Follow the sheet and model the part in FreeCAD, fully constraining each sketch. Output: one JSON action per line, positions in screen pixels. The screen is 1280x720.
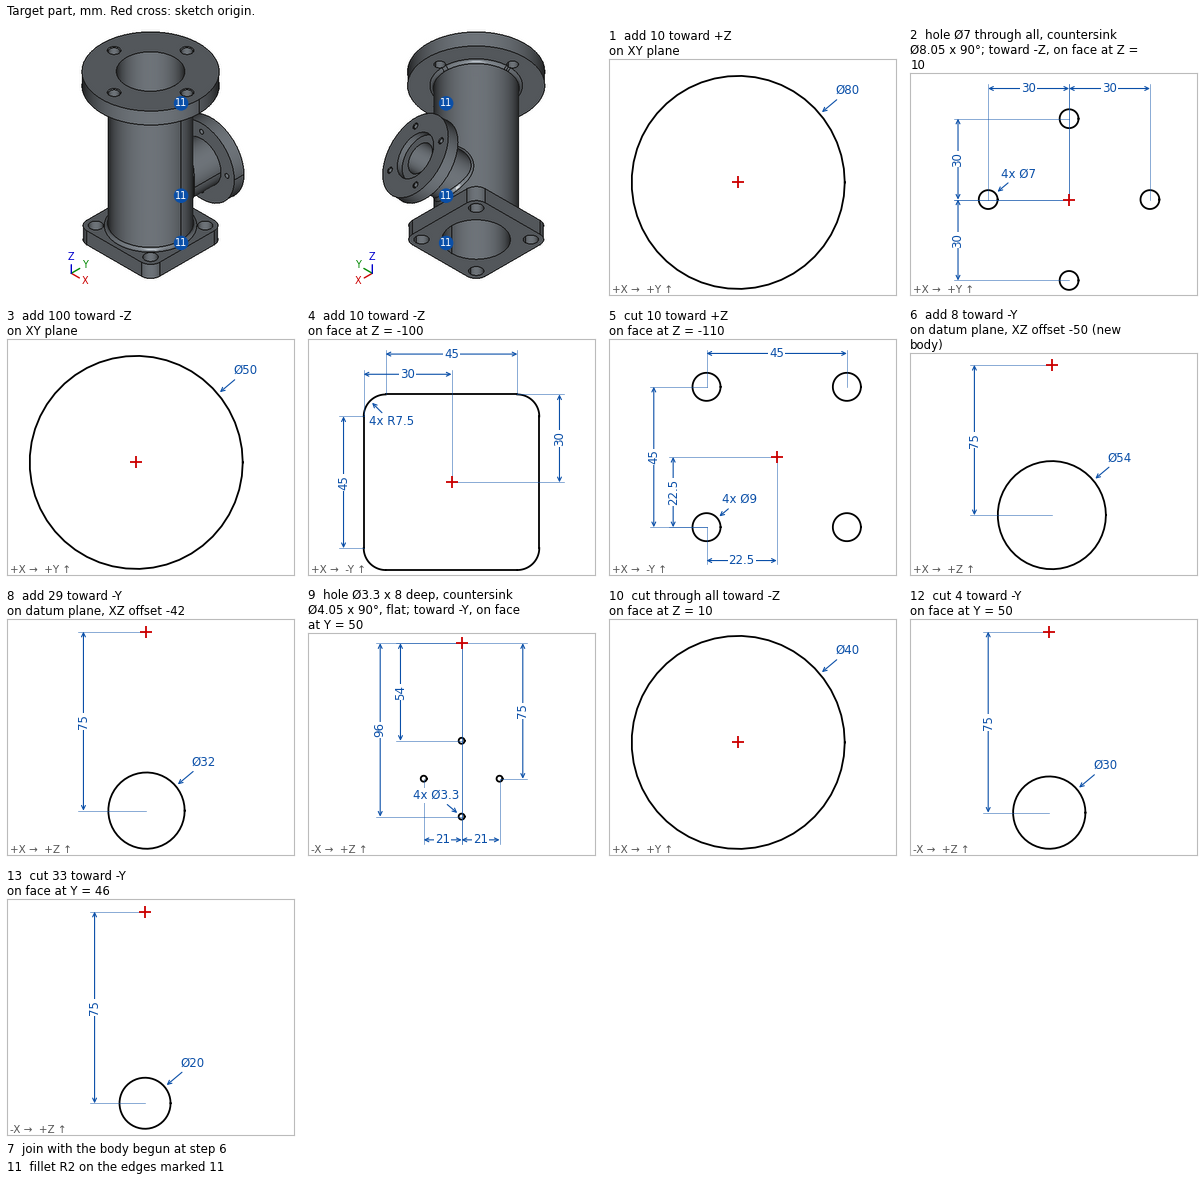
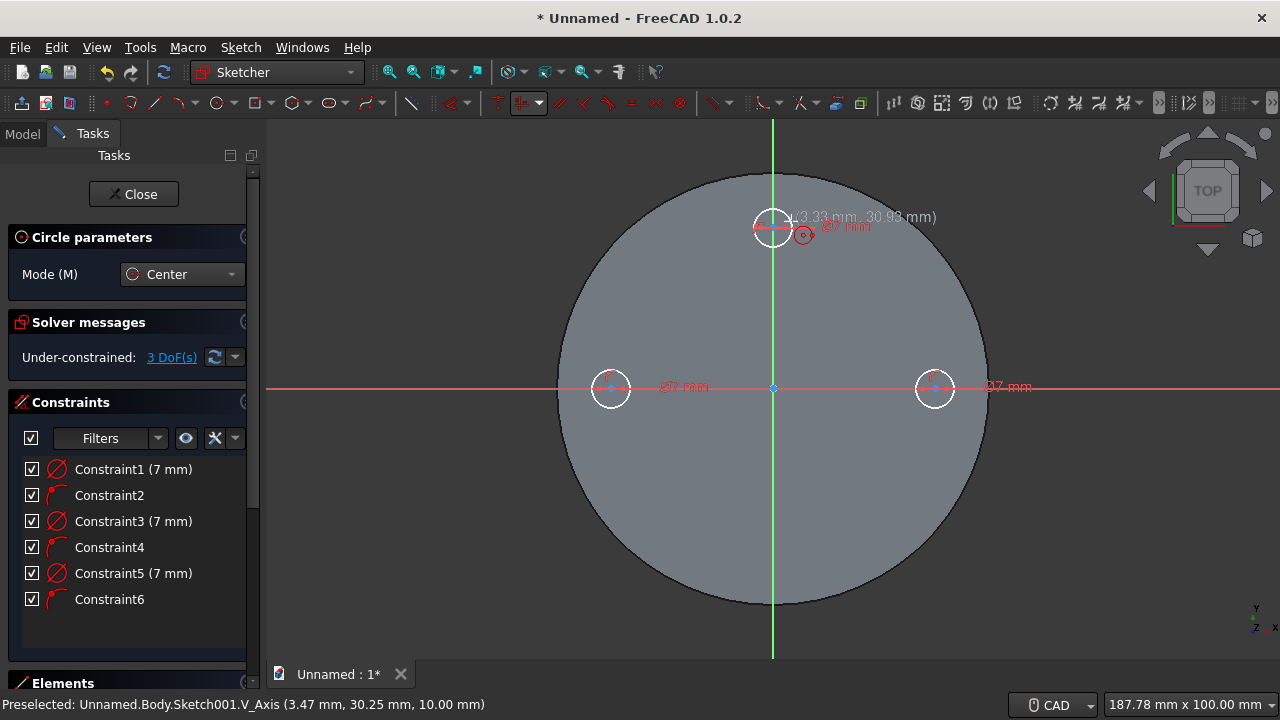
{"action": "left_click", "coordinate": [773, 551]}
{"action": "mouse_move", "coordinate": [791, 545]}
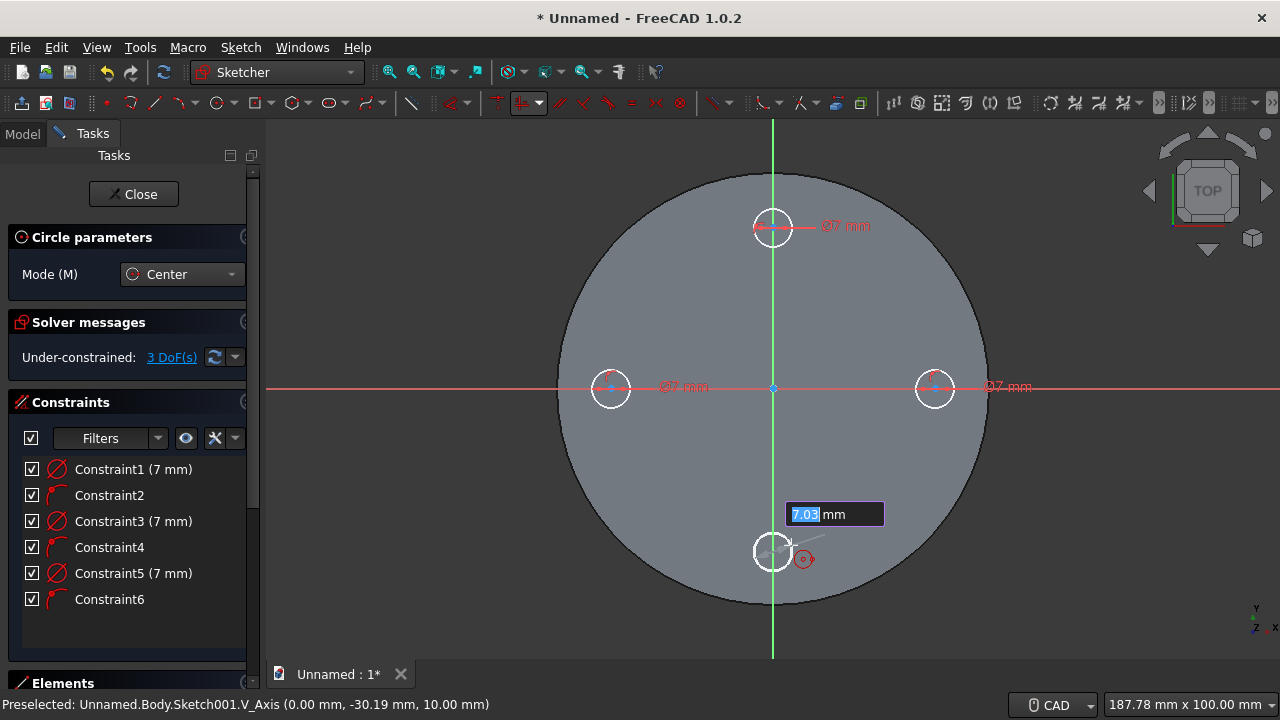
{"action": "type", "text": "7"}
{"action": "key", "text": "Return"}
{"action": "key", "text": "Escape"}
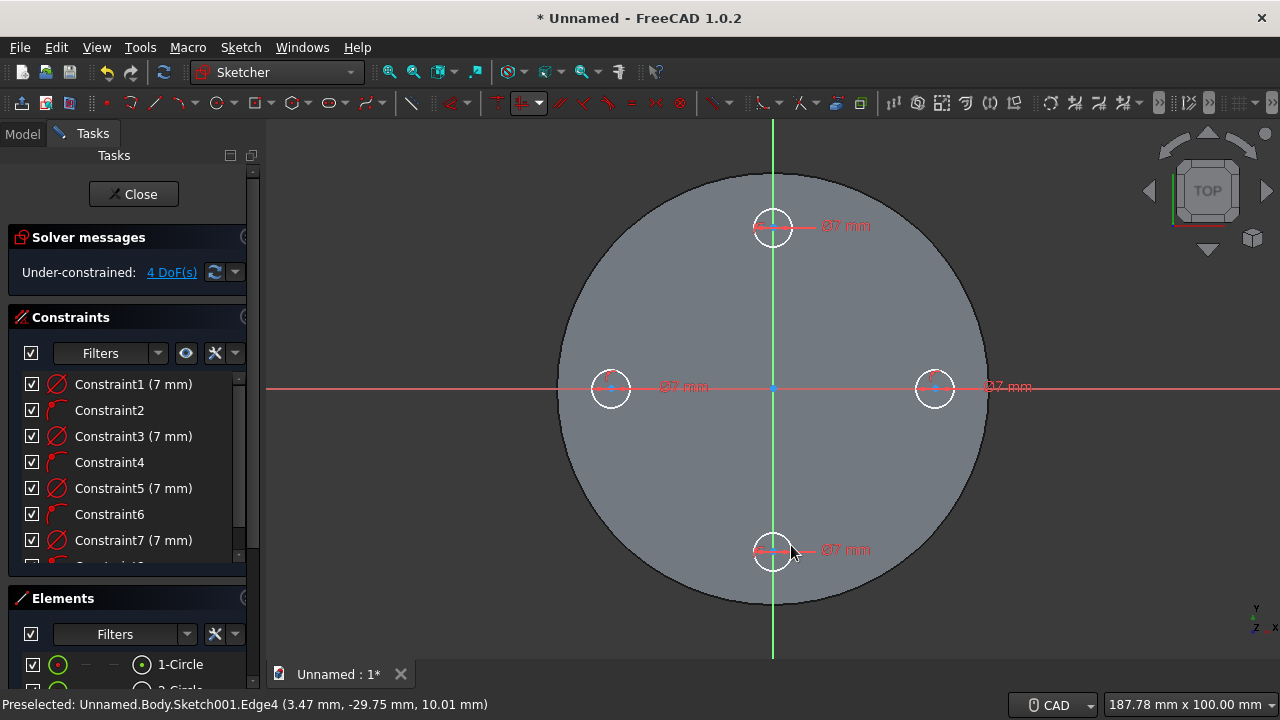
{"action": "left_click", "coordinate": [450, 104]}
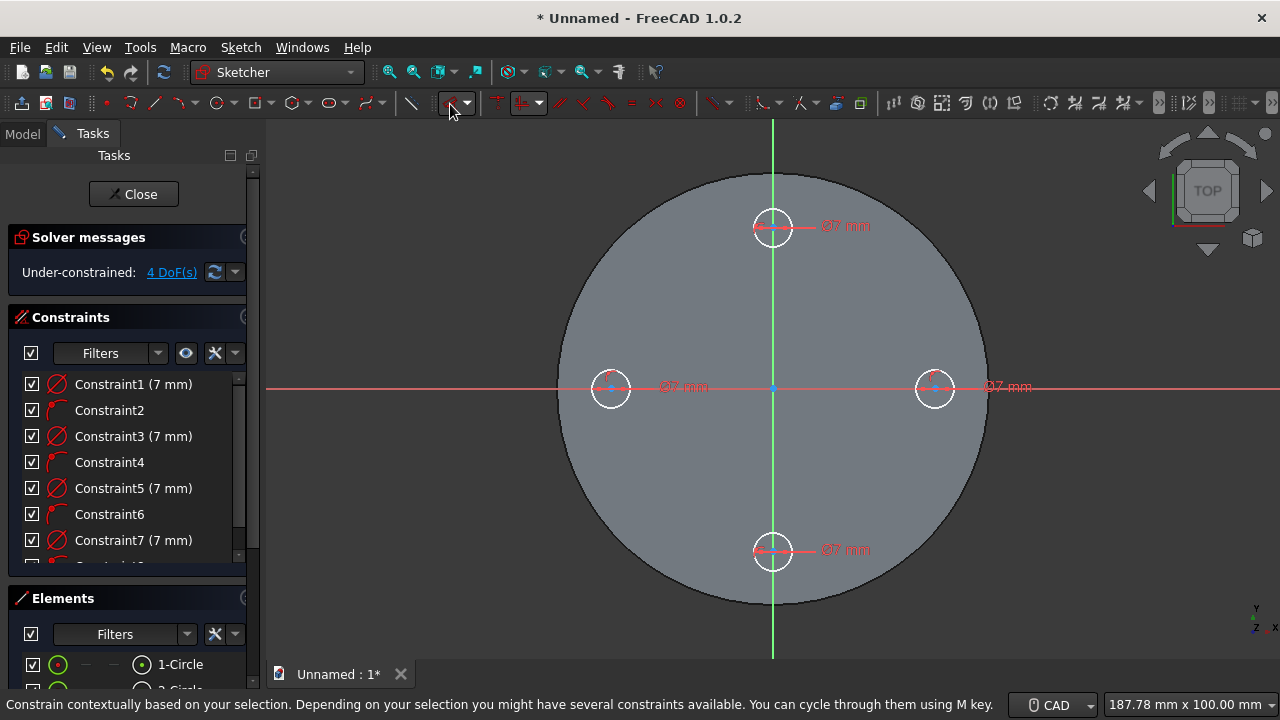
{"action": "left_click", "coordinate": [611, 389]}
{"action": "left_click", "coordinate": [692, 423]}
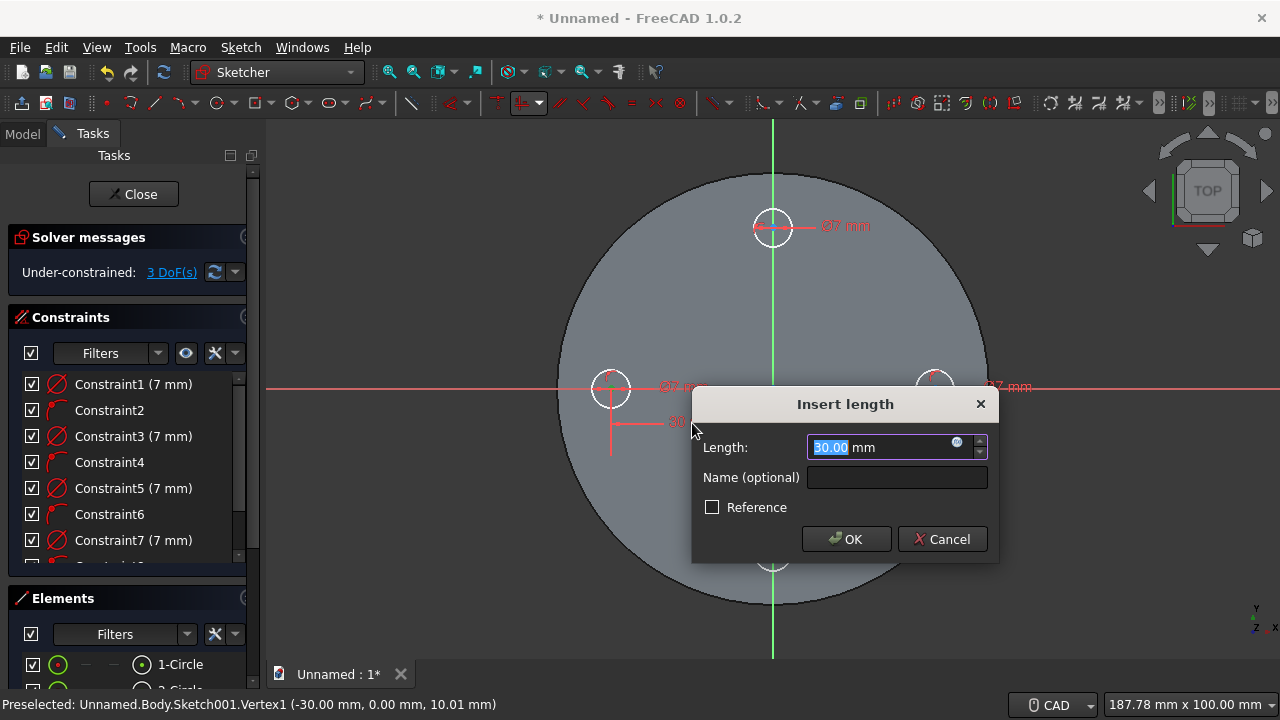
{"action": "type", "text": "30"}
{"action": "key", "text": "Return"}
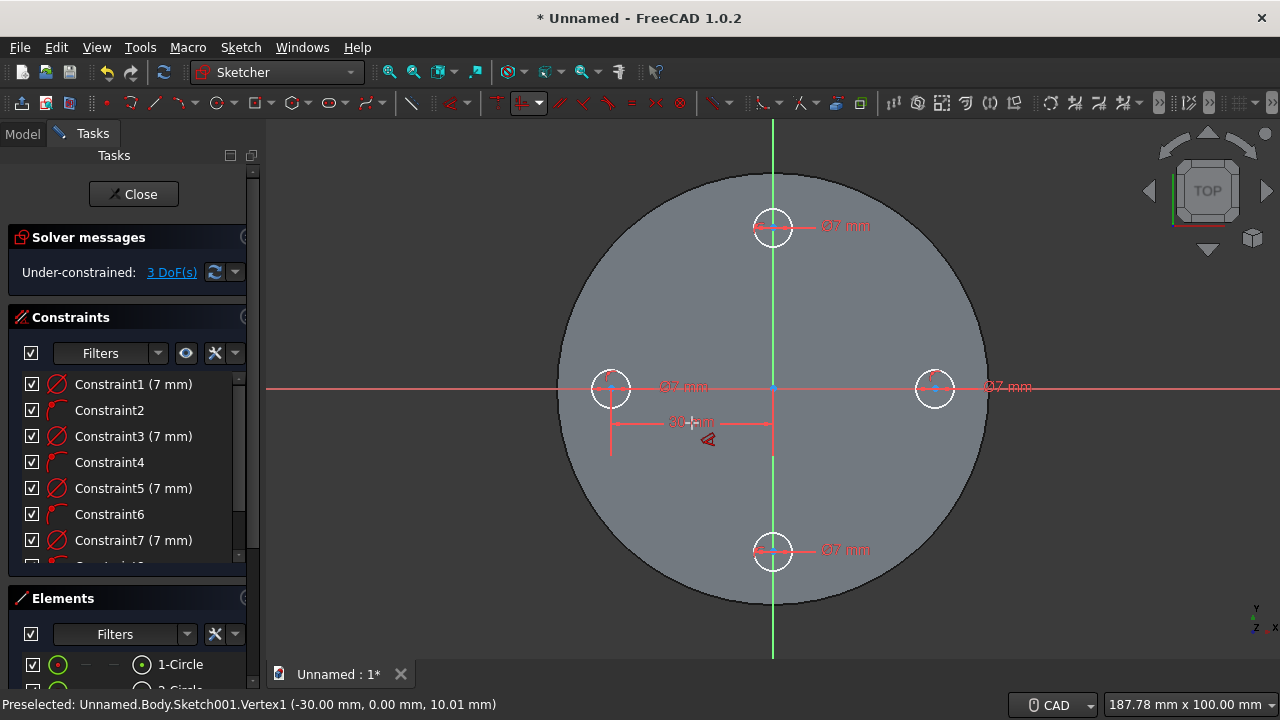
{"action": "left_click", "coordinate": [935, 389]}
{"action": "left_click", "coordinate": [854, 423]}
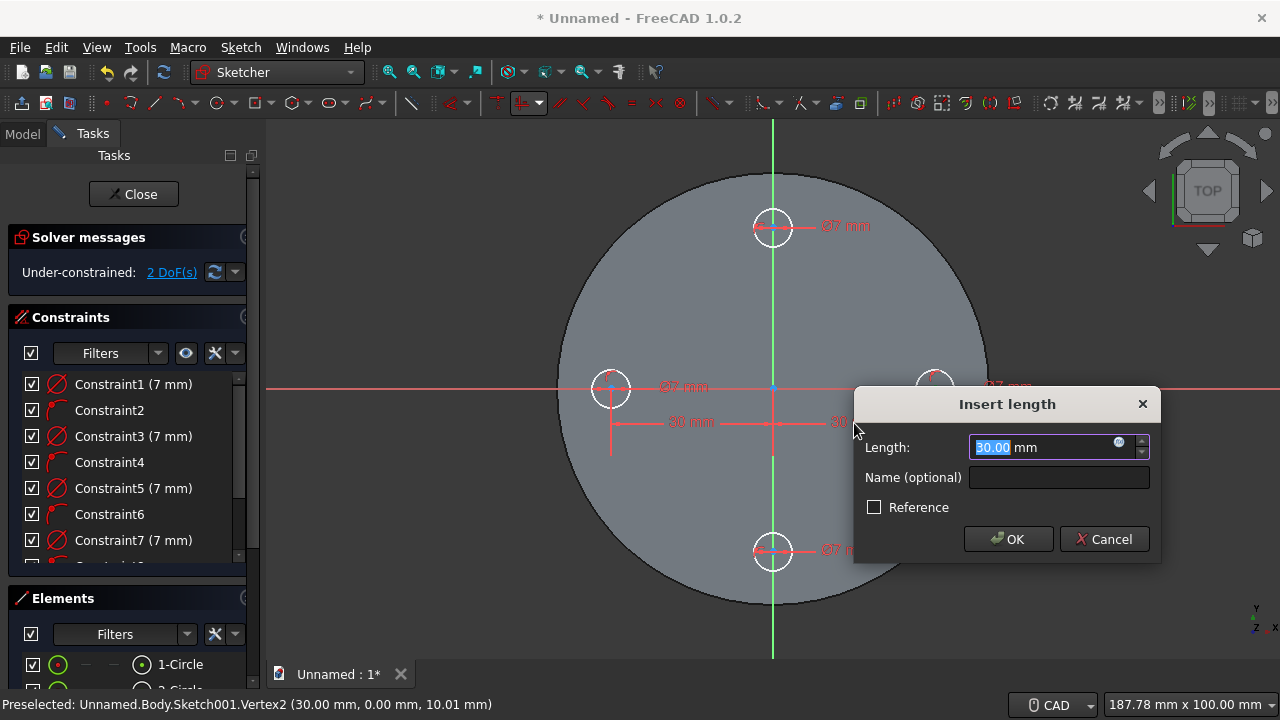
{"action": "type", "text": "30"}
{"action": "key", "text": "Return"}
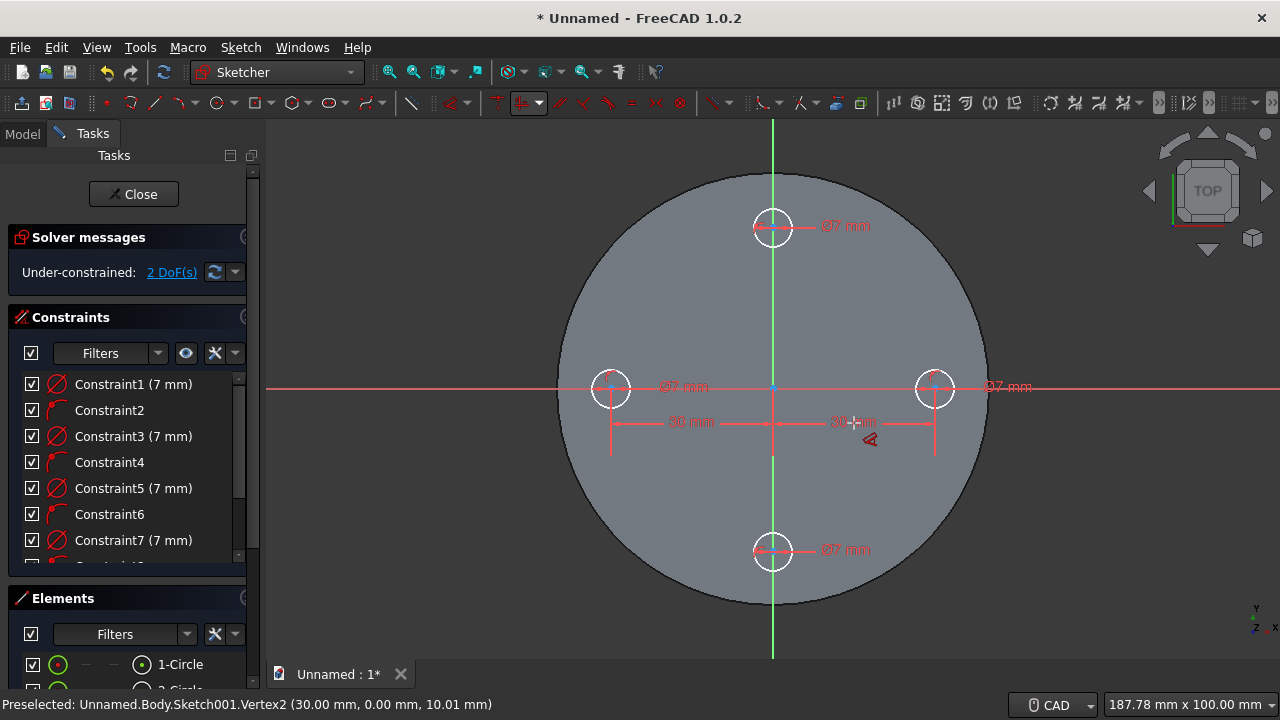
{"action": "left_click", "coordinate": [773, 228]}
{"action": "left_click", "coordinate": [807, 308]}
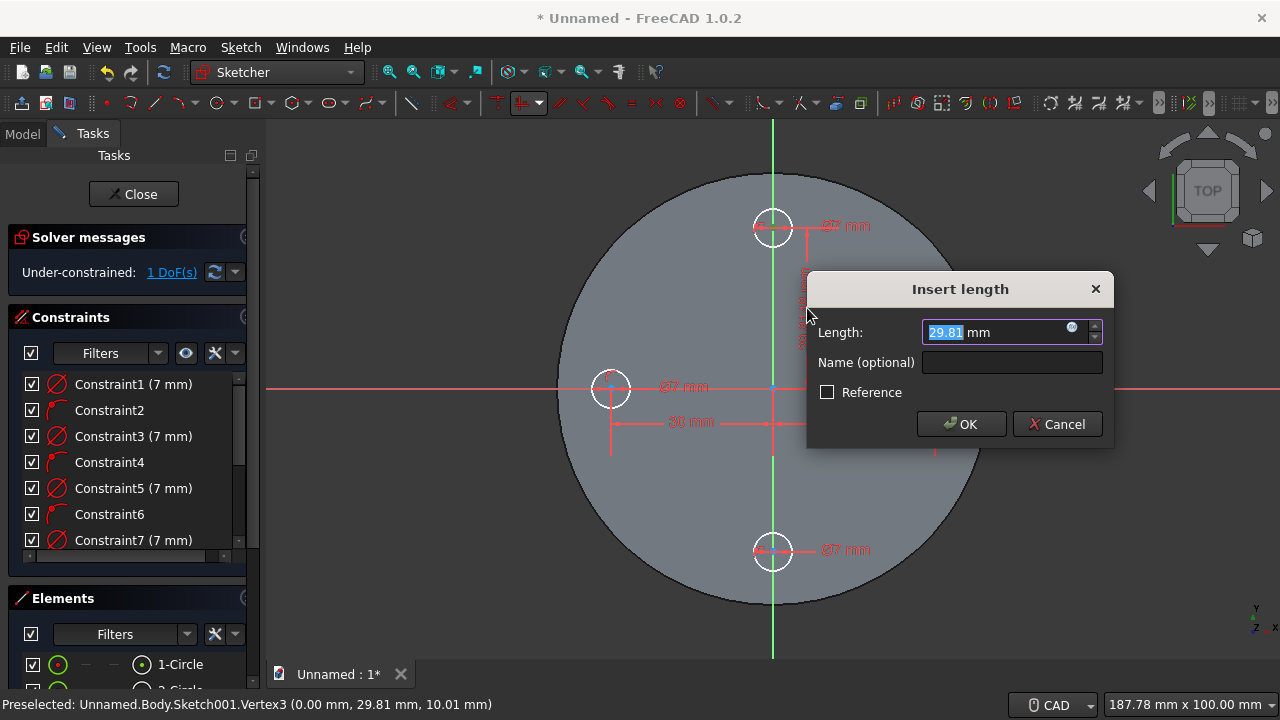
{"action": "type", "text": "30"}
{"action": "key", "text": "Return"}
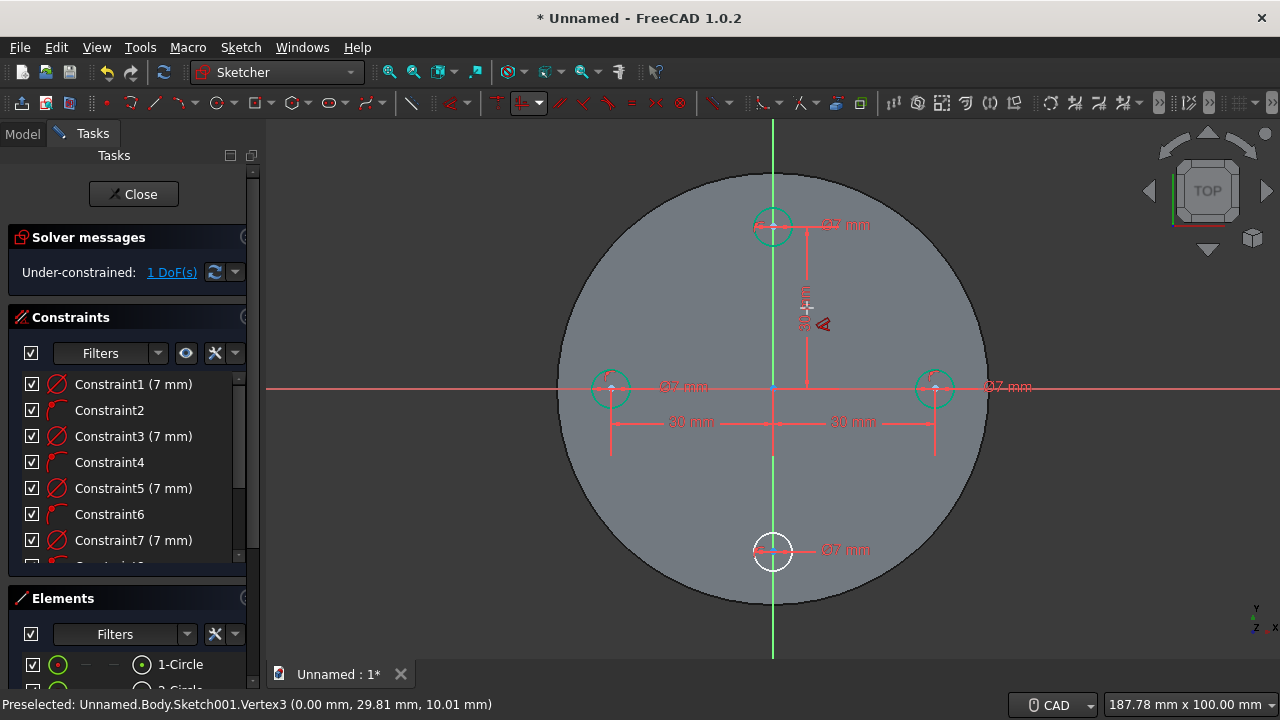
{"action": "left_click", "coordinate": [773, 552]}
{"action": "left_click", "coordinate": [807, 470]}